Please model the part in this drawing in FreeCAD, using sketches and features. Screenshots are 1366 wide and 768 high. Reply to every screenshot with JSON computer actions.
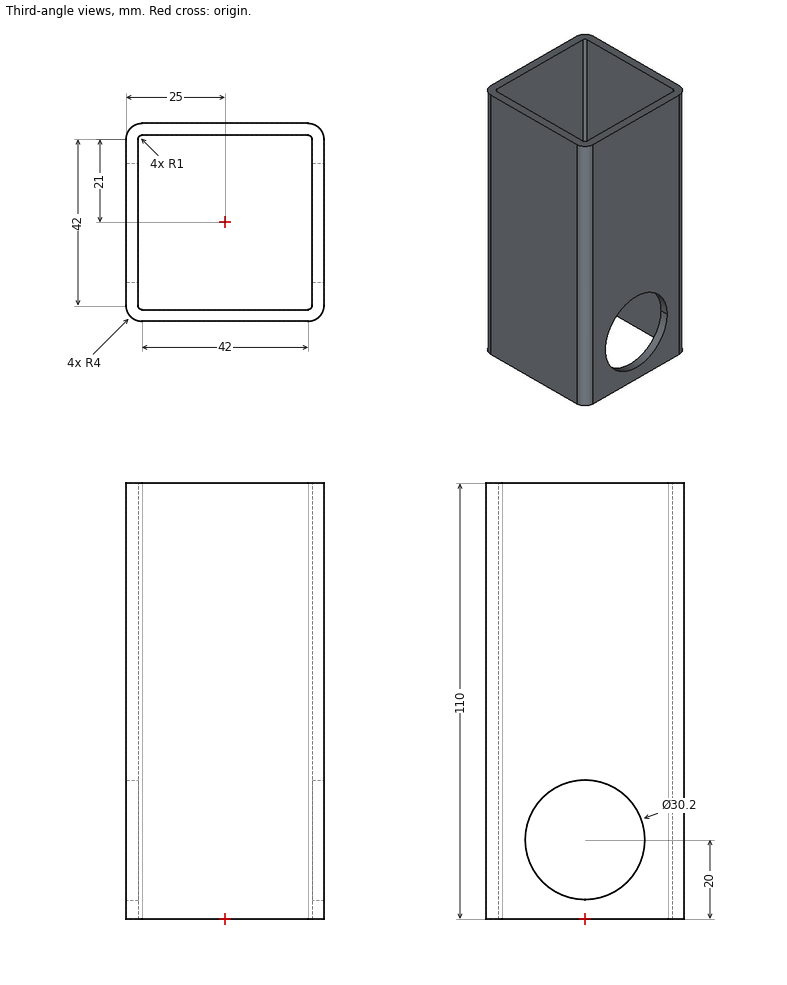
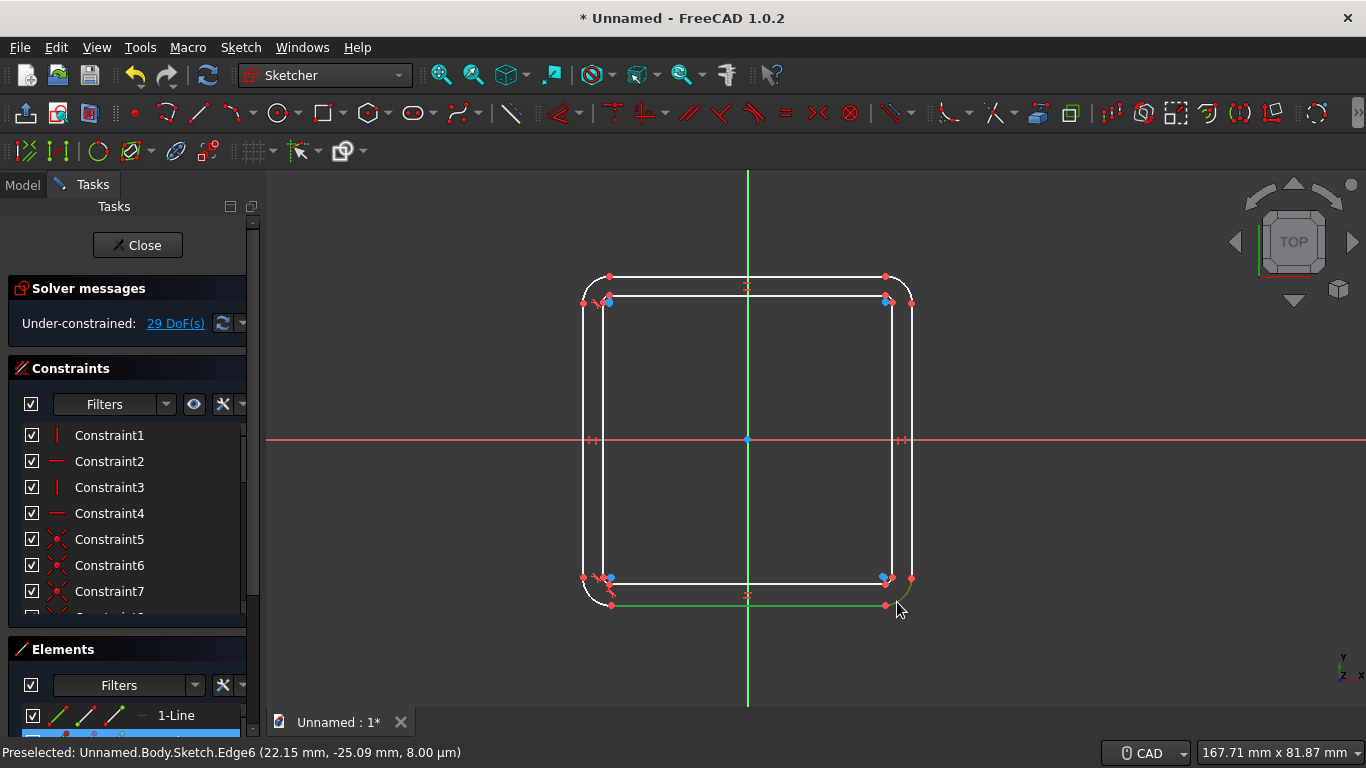
{"action": "key", "text": "t"}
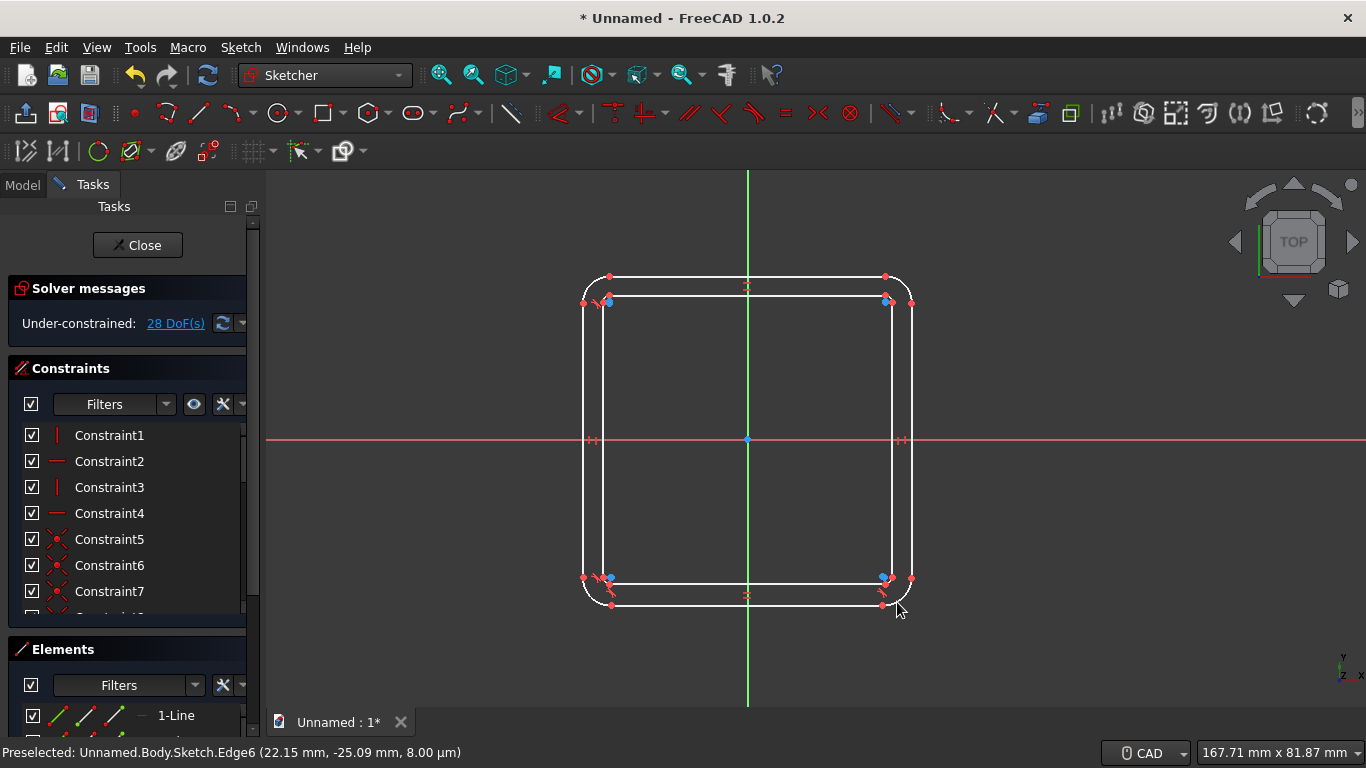
{"action": "left_click", "coordinate": [912, 496]}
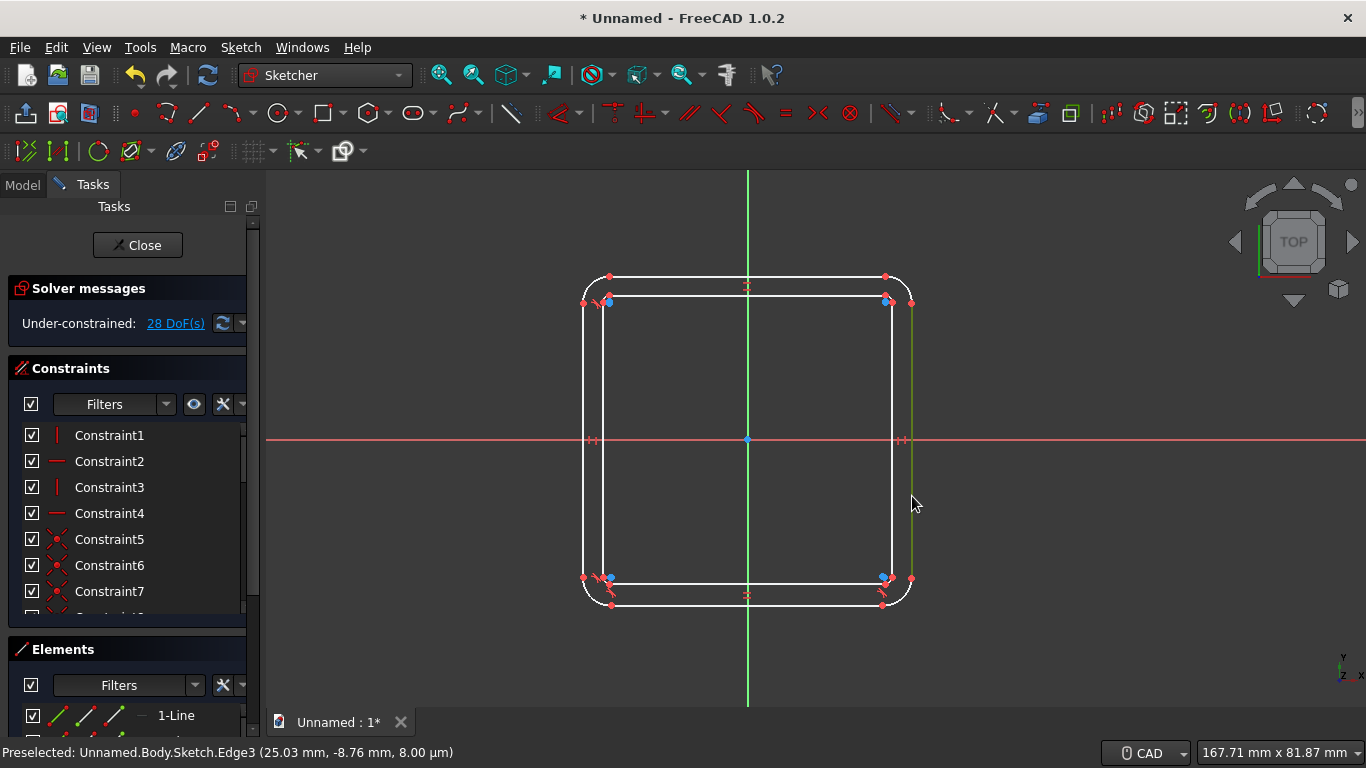
{"action": "left_click", "coordinate": [896, 603]}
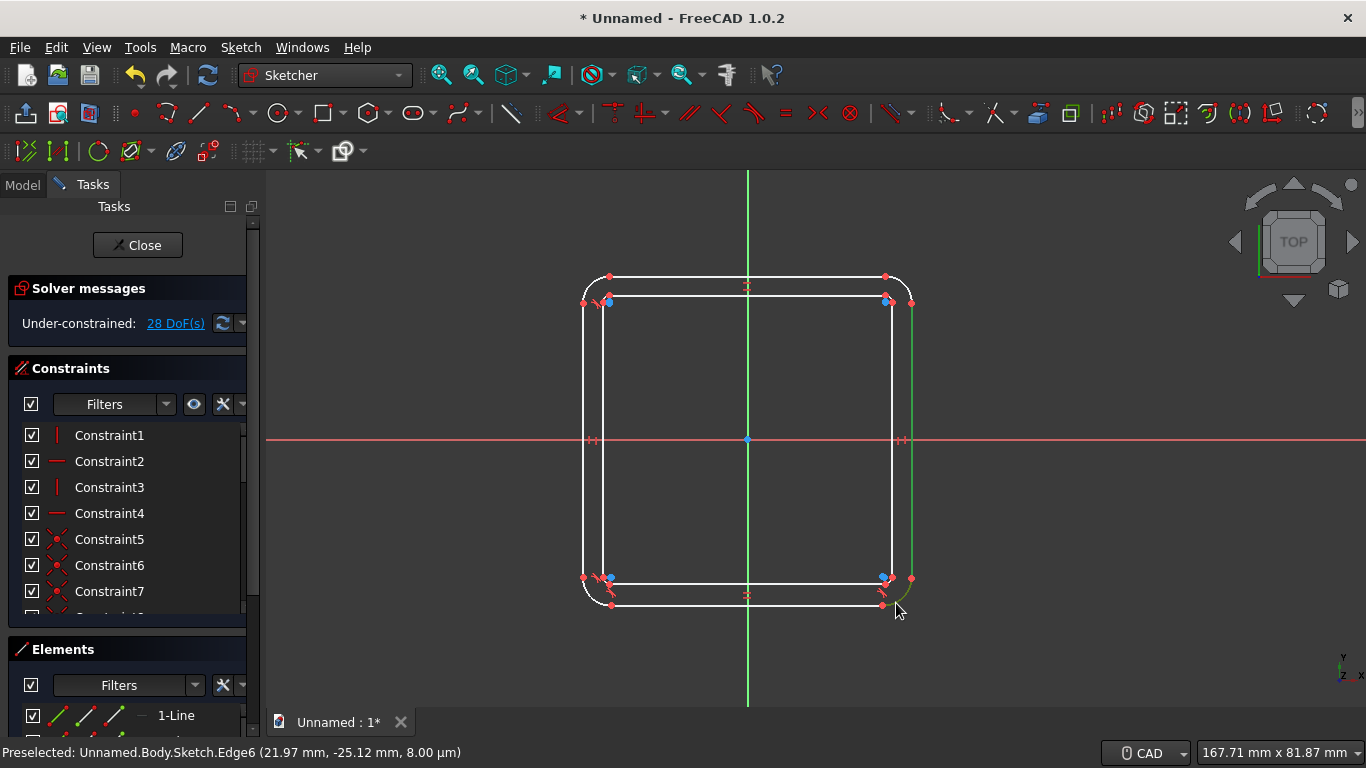
{"action": "left_click", "coordinate": [754, 114]}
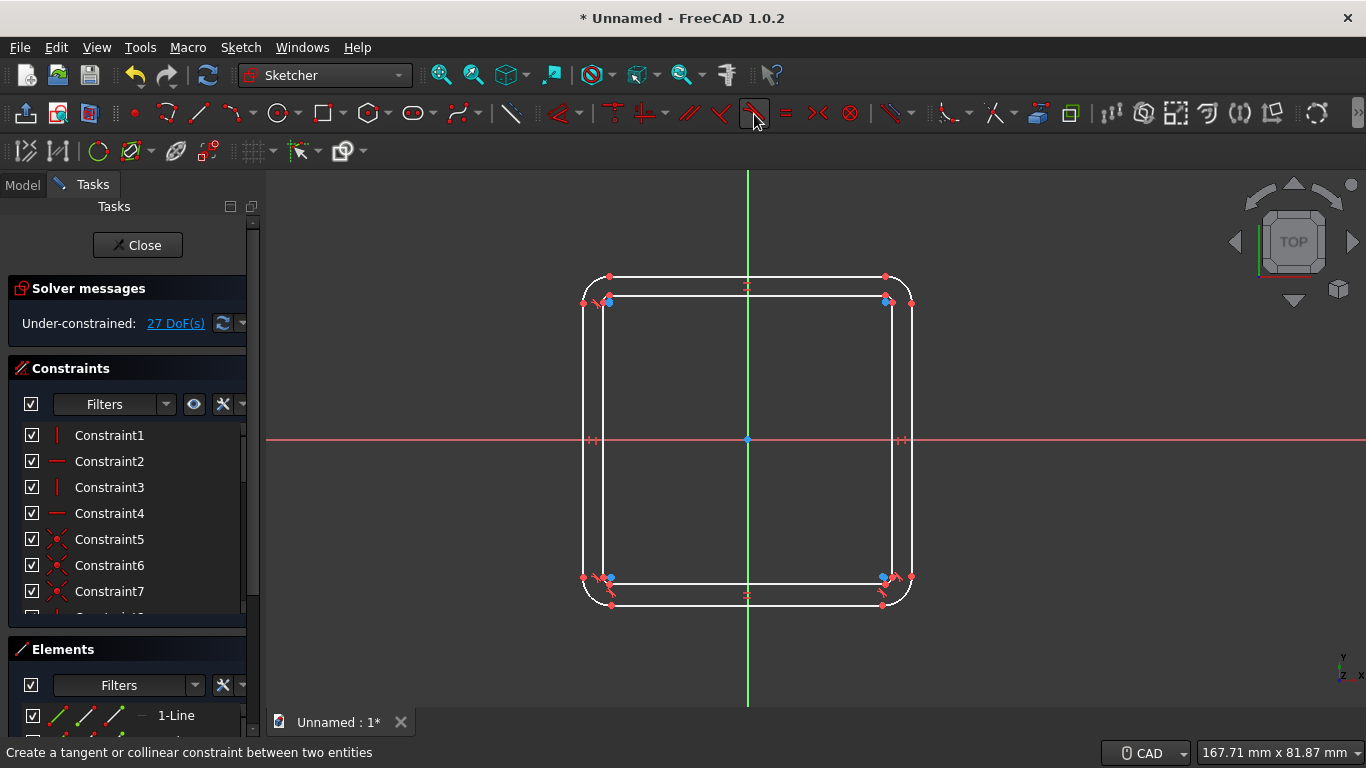
{"action": "left_click", "coordinate": [912, 495]}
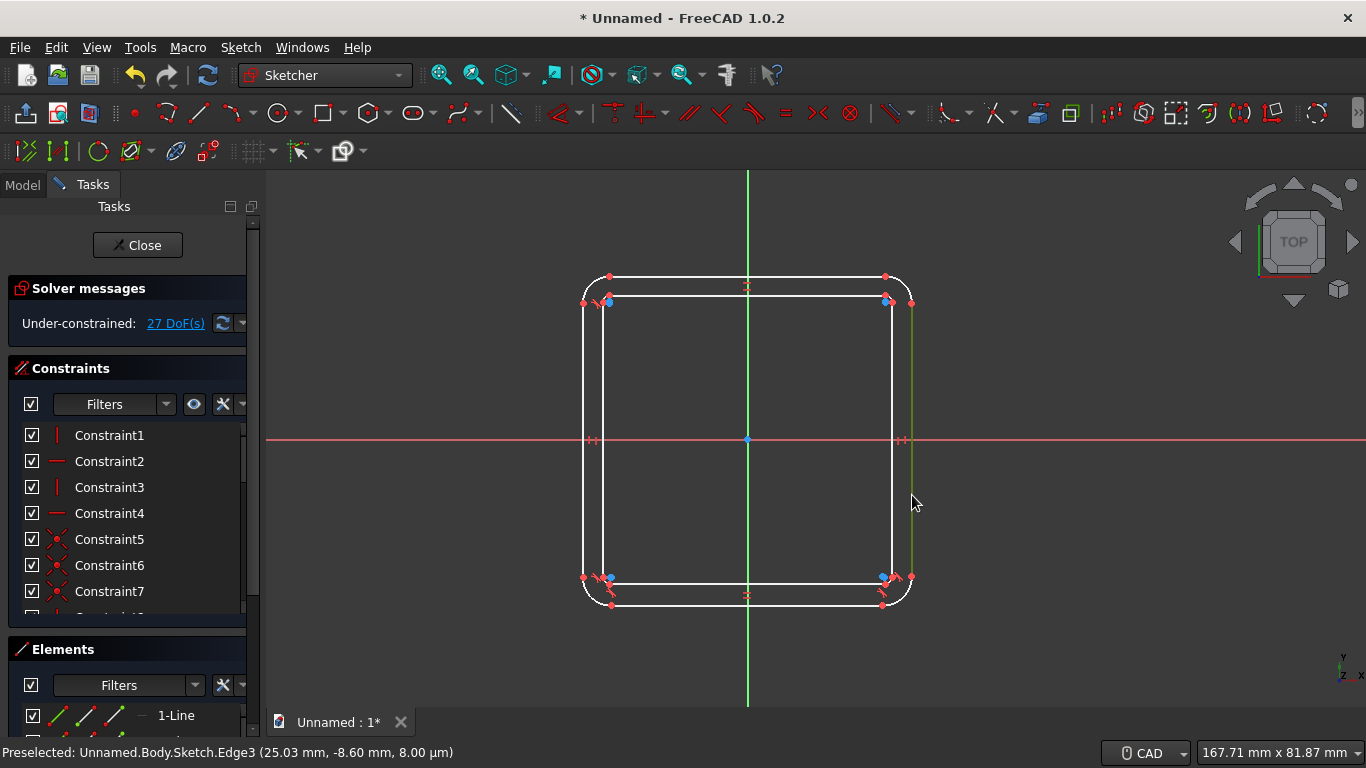
{"action": "left_click", "coordinate": [909, 291]}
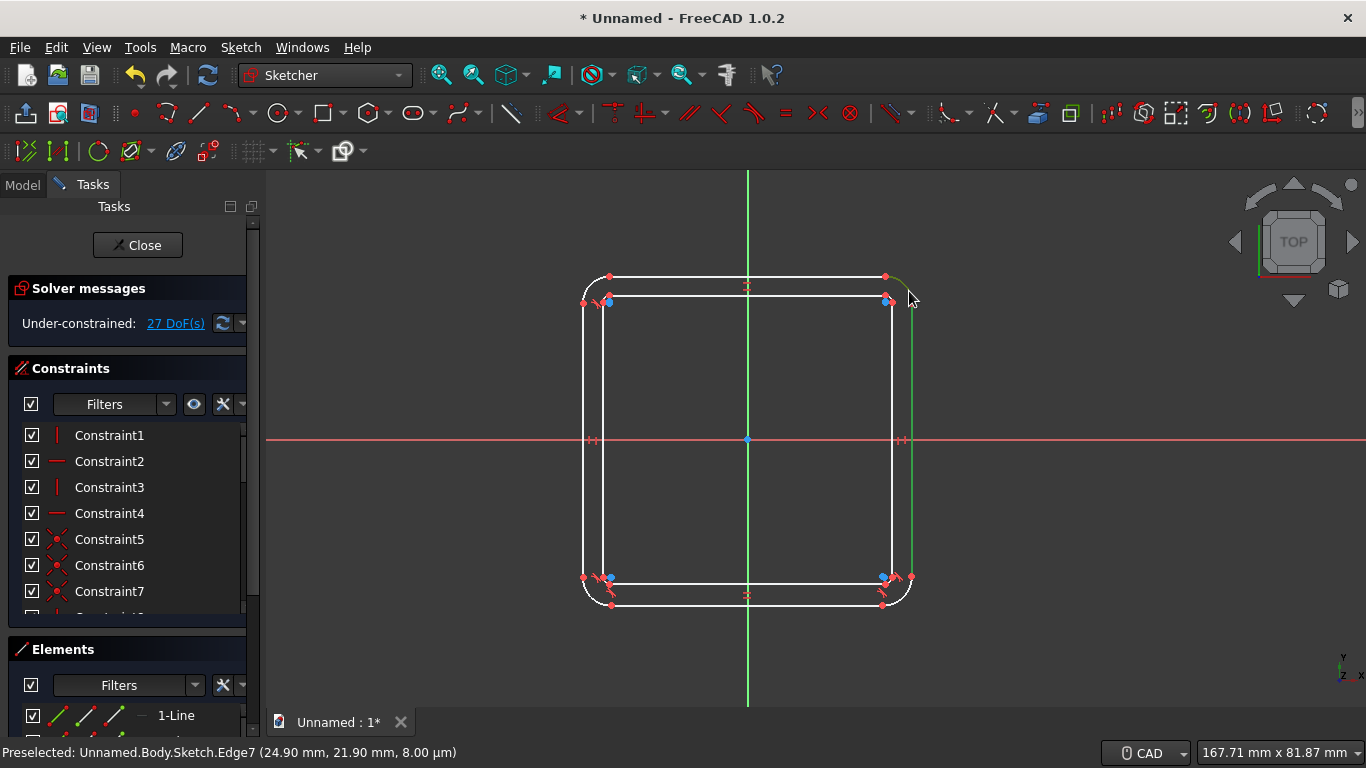
{"action": "left_click", "coordinate": [754, 114]}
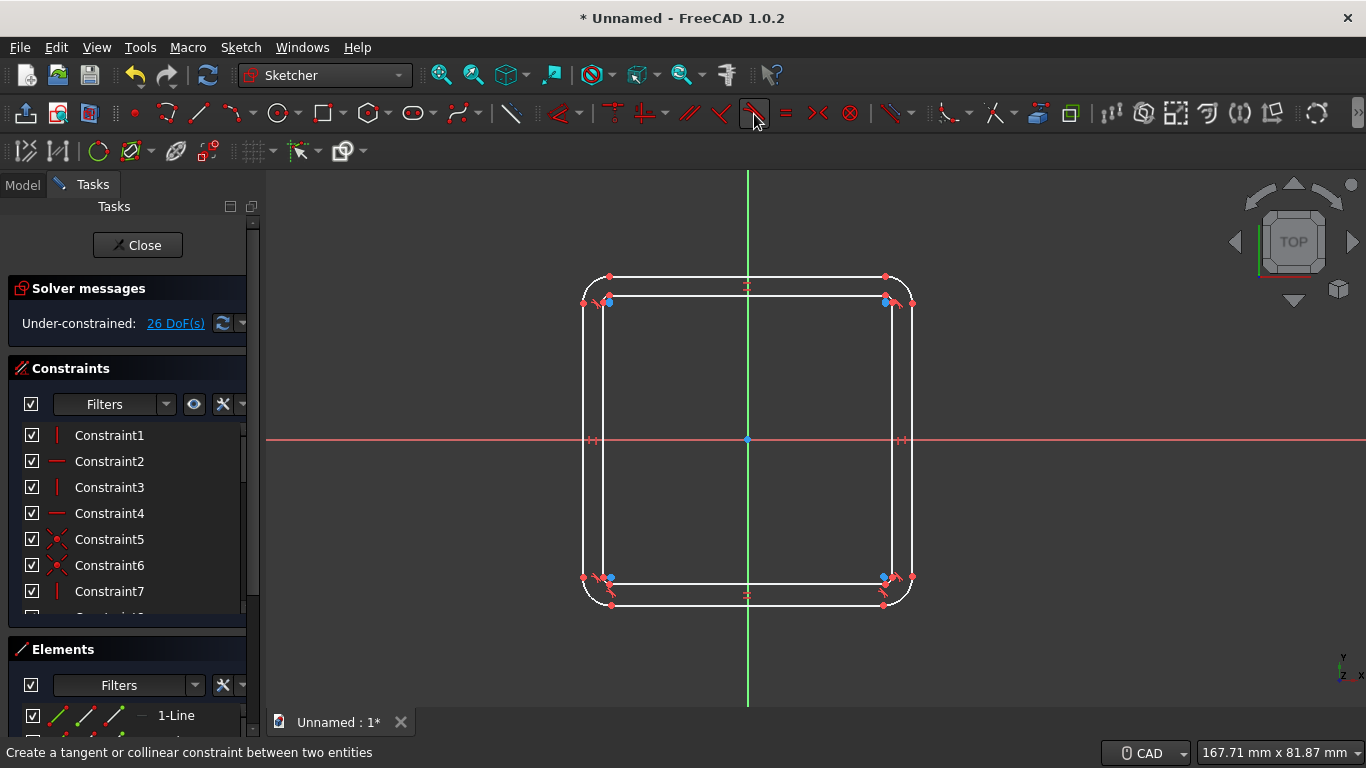
{"action": "left_click", "coordinate": [803, 277]}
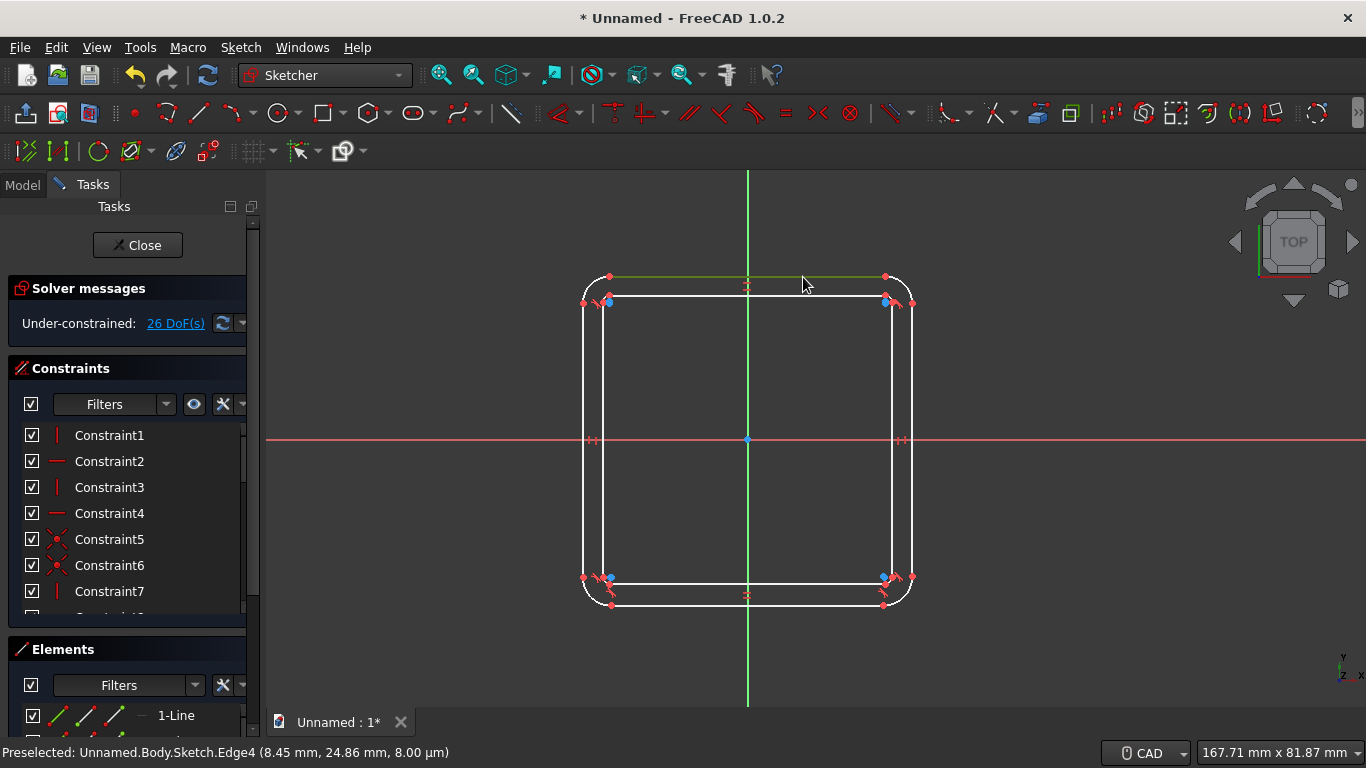
{"action": "left_click", "coordinate": [909, 291]}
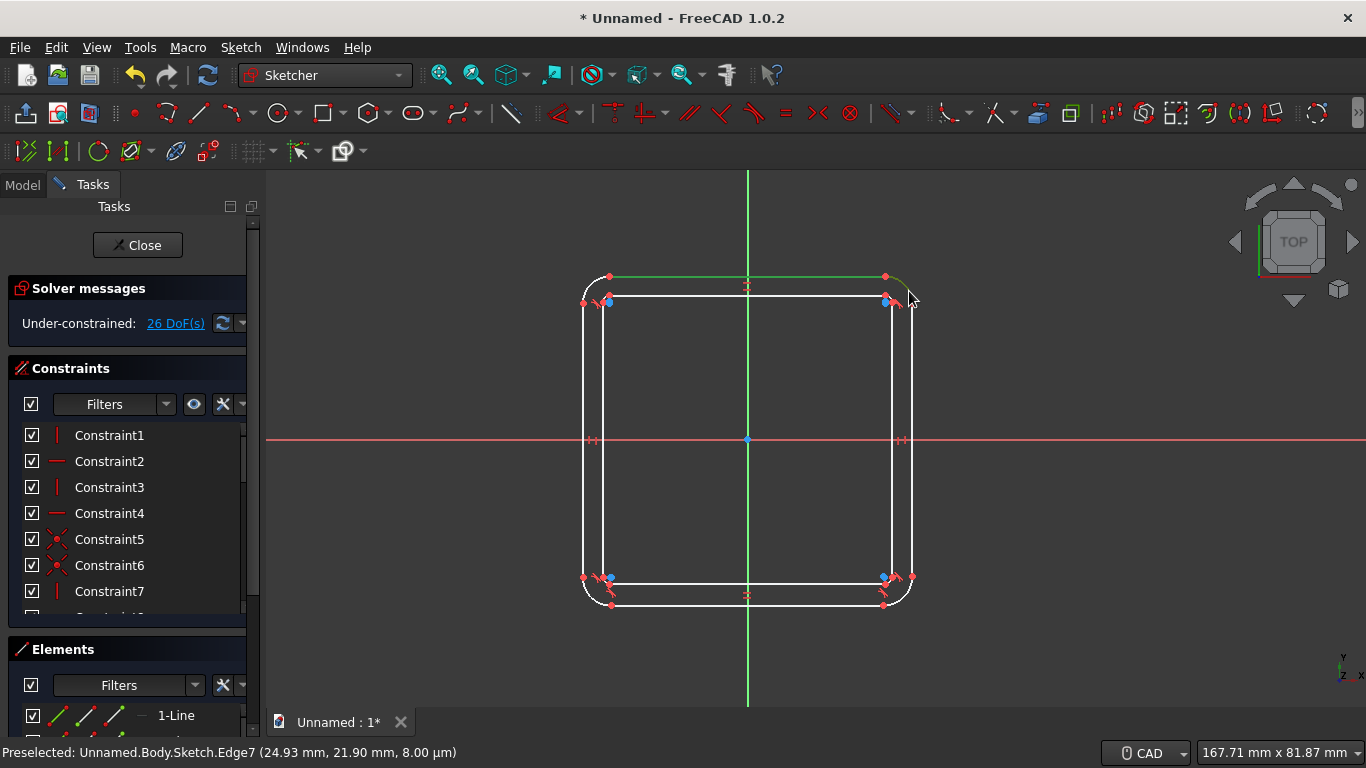
{"action": "left_click", "coordinate": [754, 114]}